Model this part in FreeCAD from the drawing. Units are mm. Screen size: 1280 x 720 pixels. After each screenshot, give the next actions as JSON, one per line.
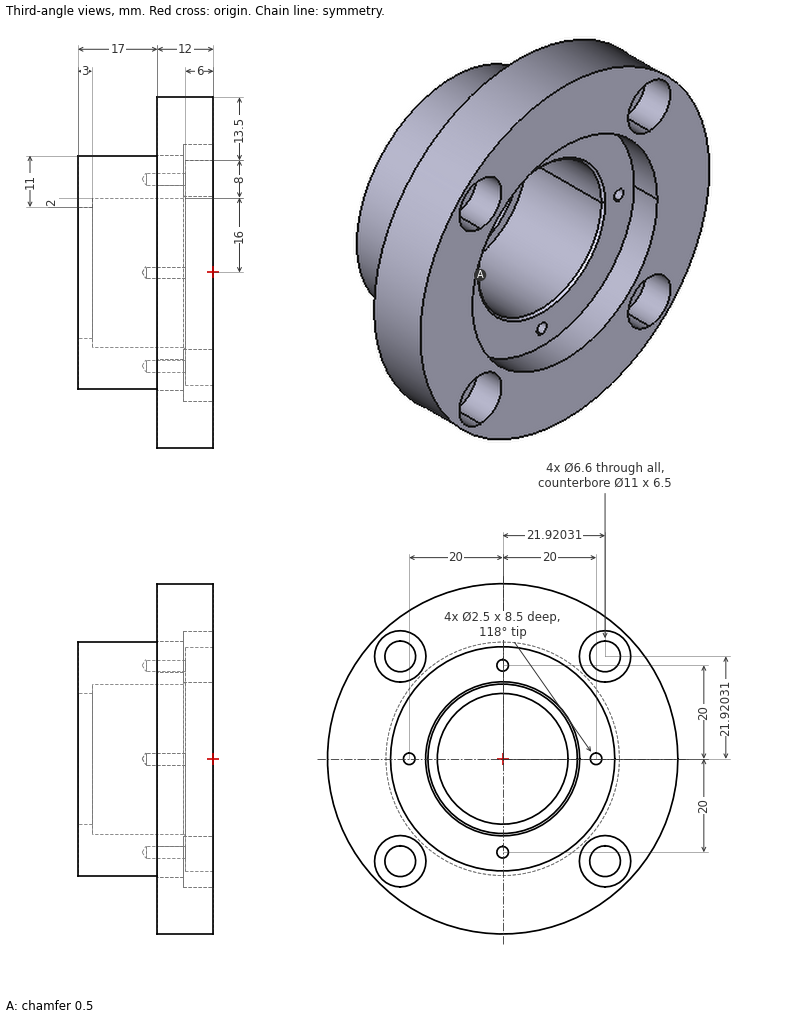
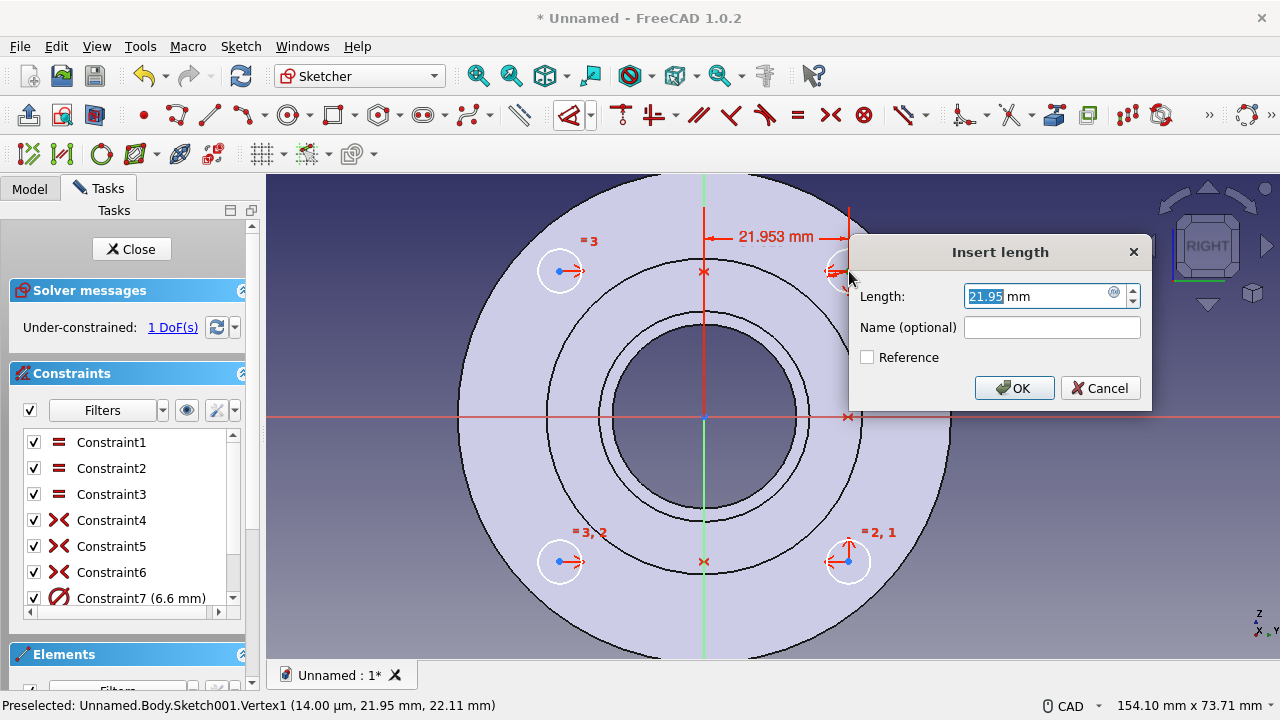
{"action": "type", "text": "21.92031"}
{"action": "key", "text": "Return"}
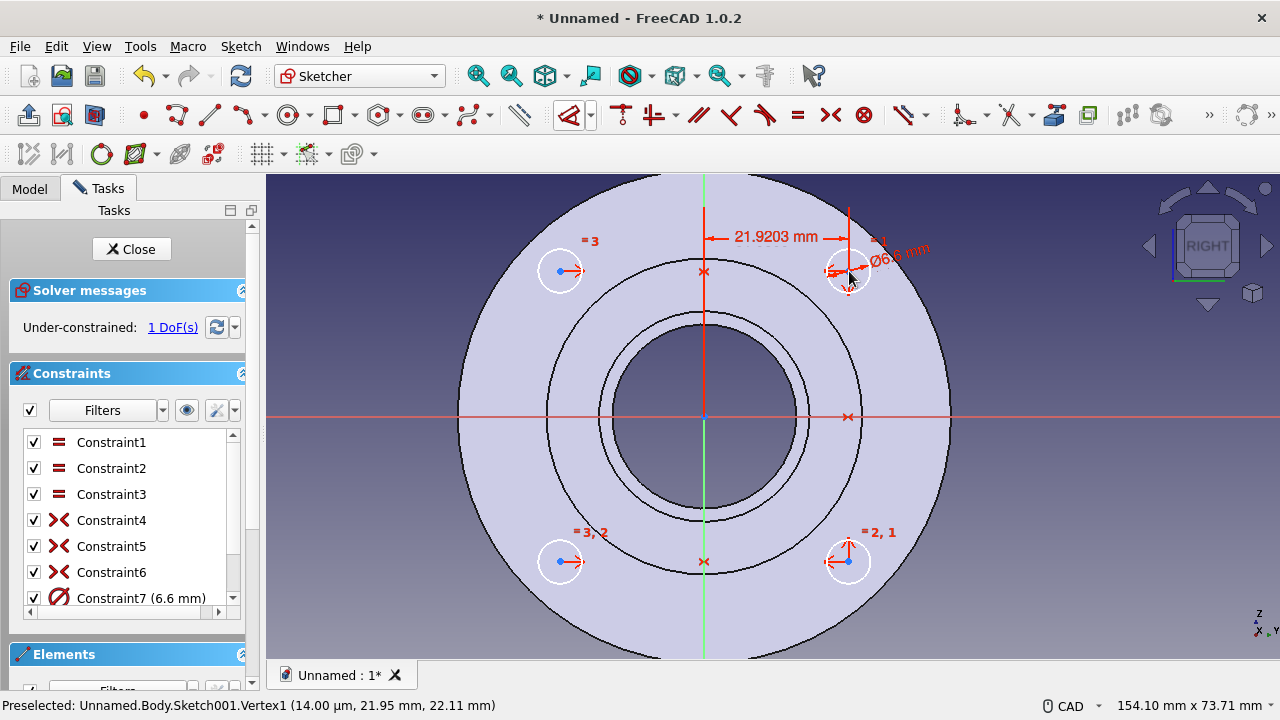
{"action": "left_click", "coordinate": [849, 271]}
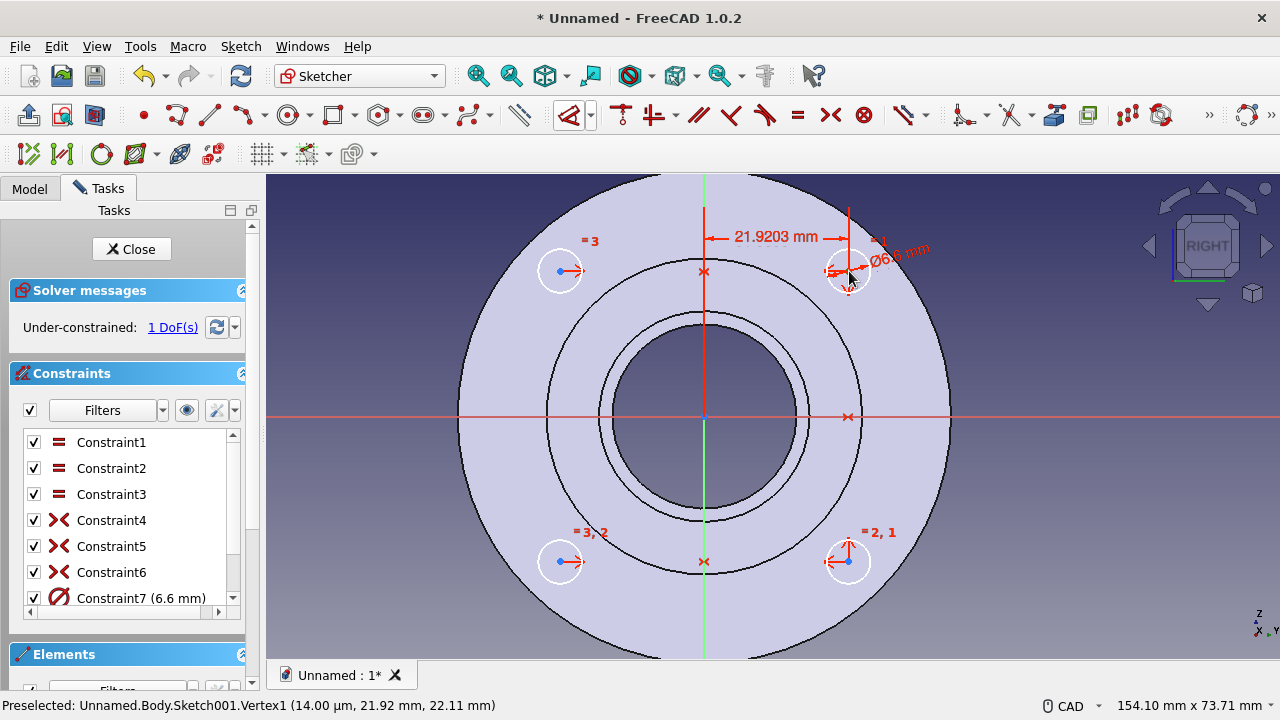
{"action": "key", "text": "i"}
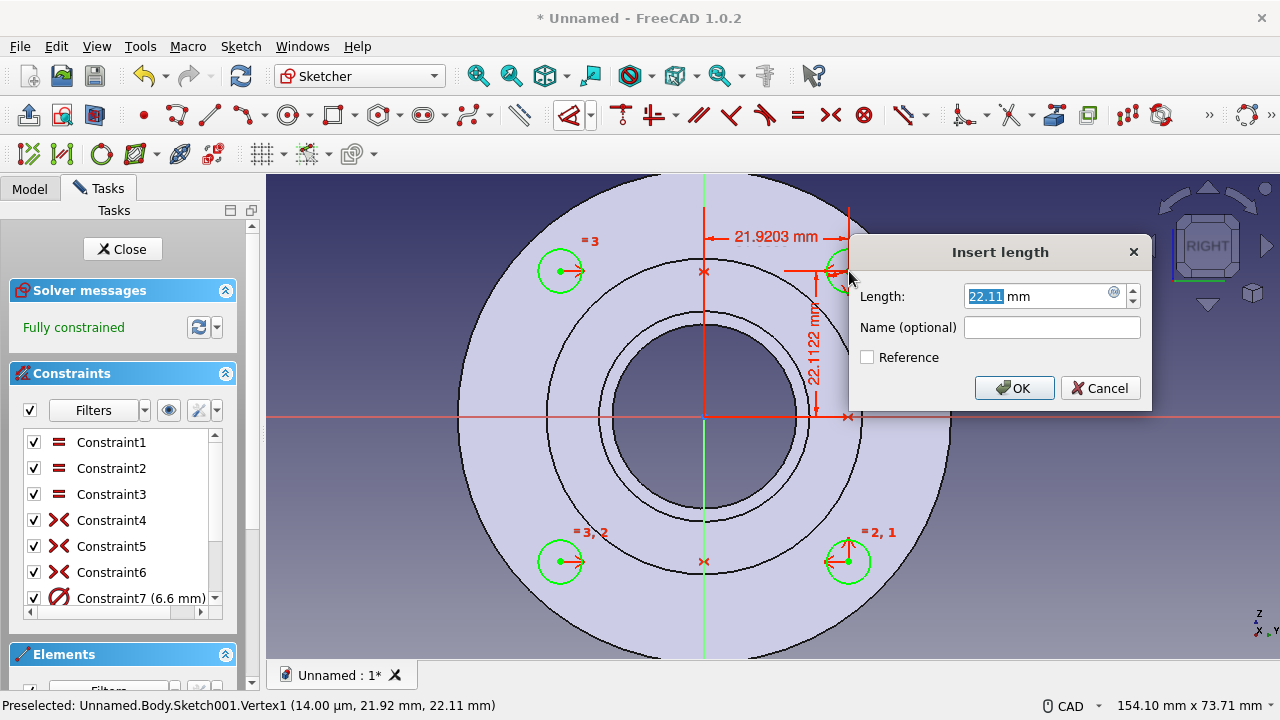
{"action": "type", "text": "21.92031"}
{"action": "key", "text": "Return"}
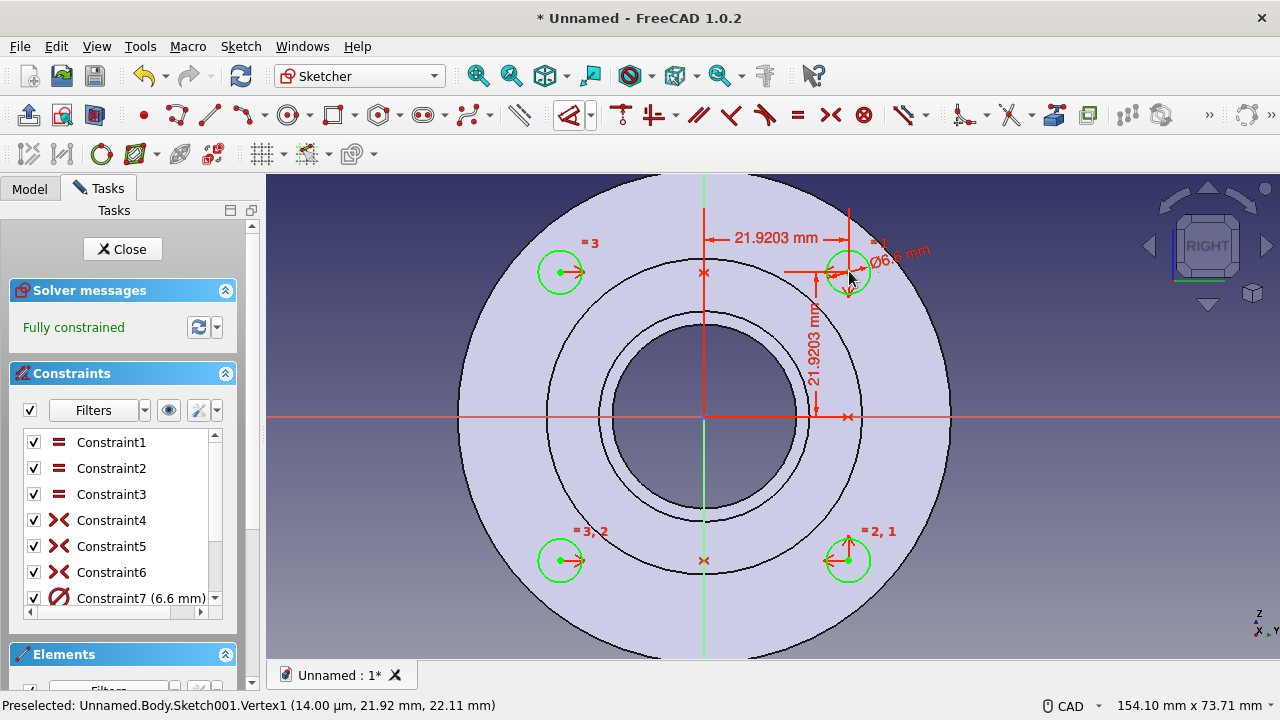
{"action": "left_click", "coordinate": [123, 249]}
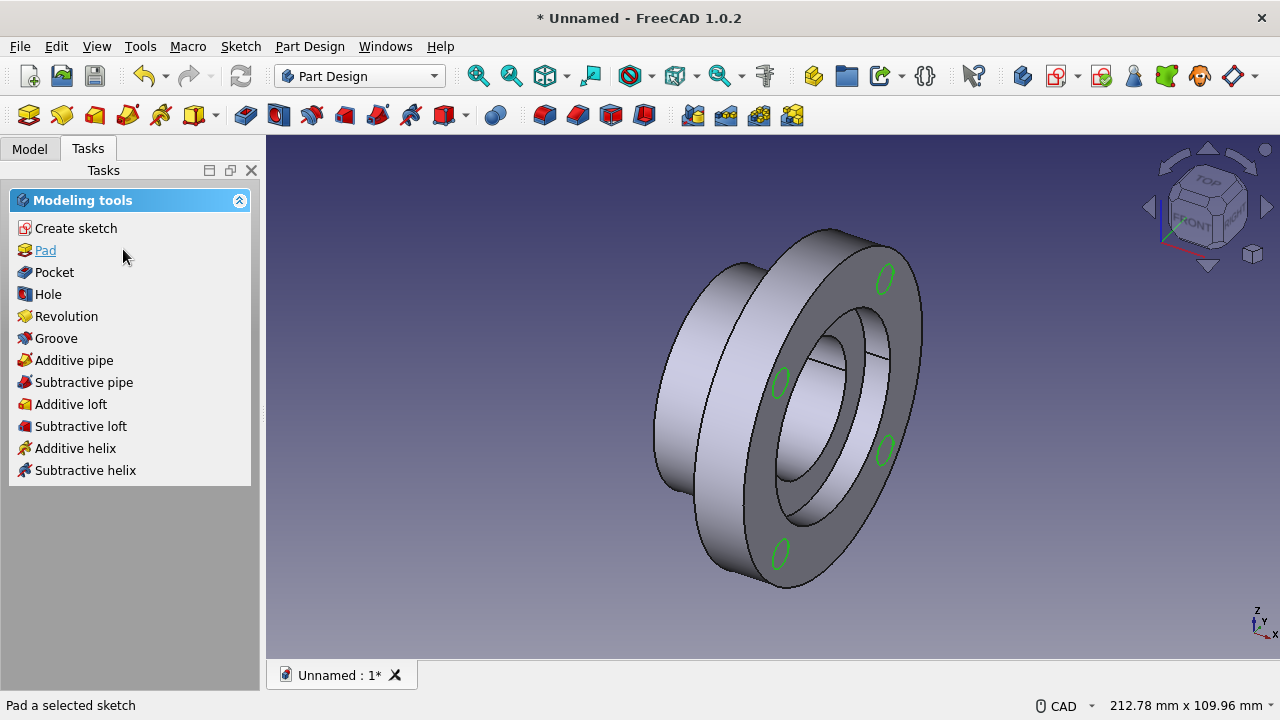
{"action": "left_click", "coordinate": [279, 116]}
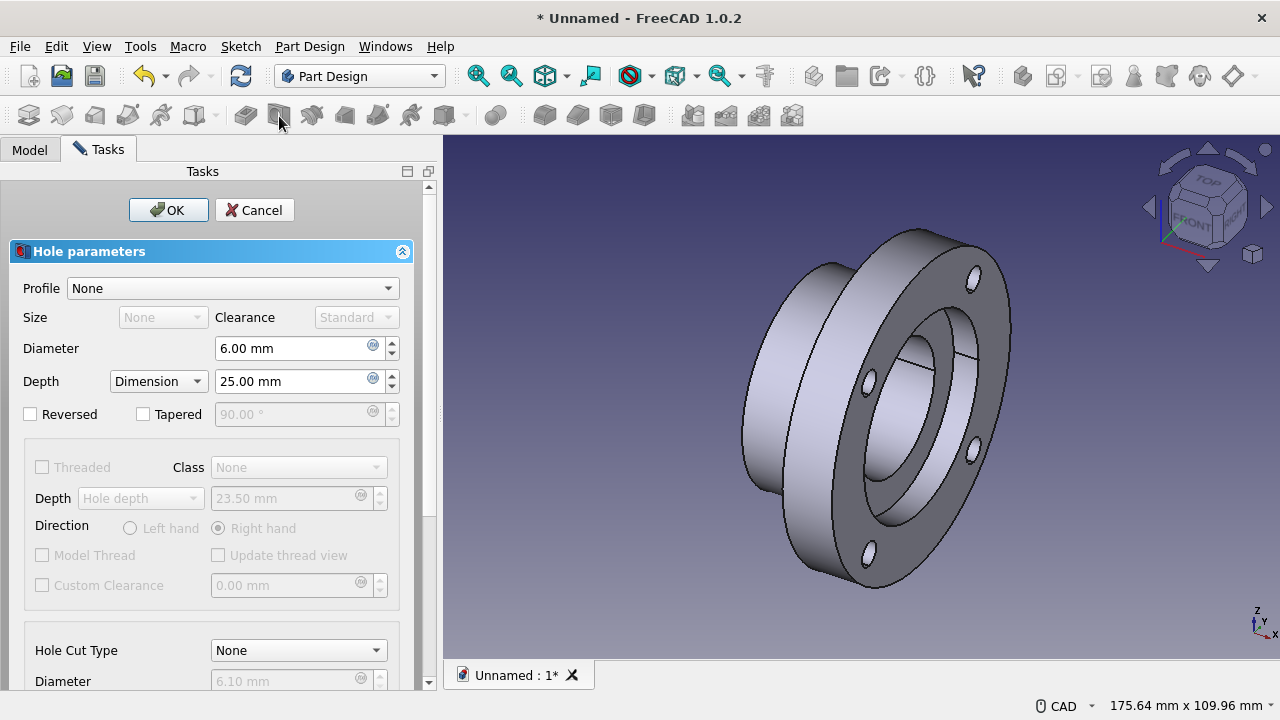
{"action": "triple_click", "coordinate": [300, 348]}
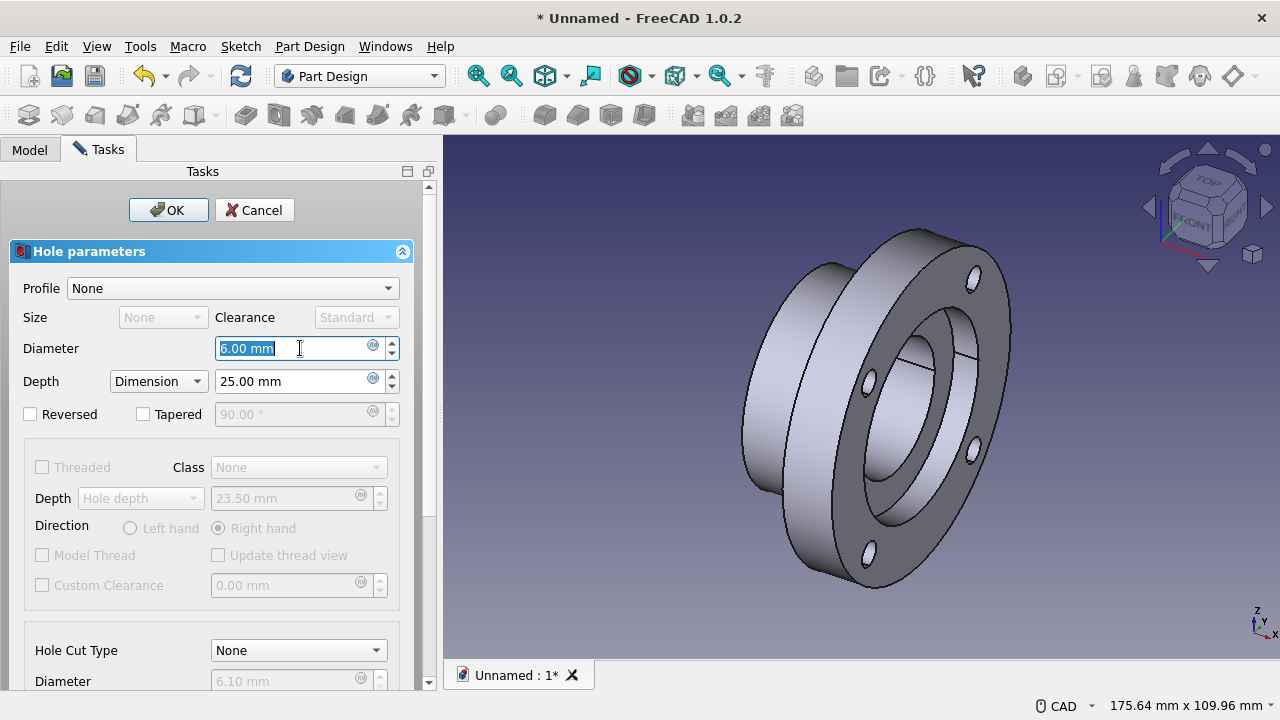
{"action": "type", "text": "6.6"}
{"action": "key", "text": "Tab"}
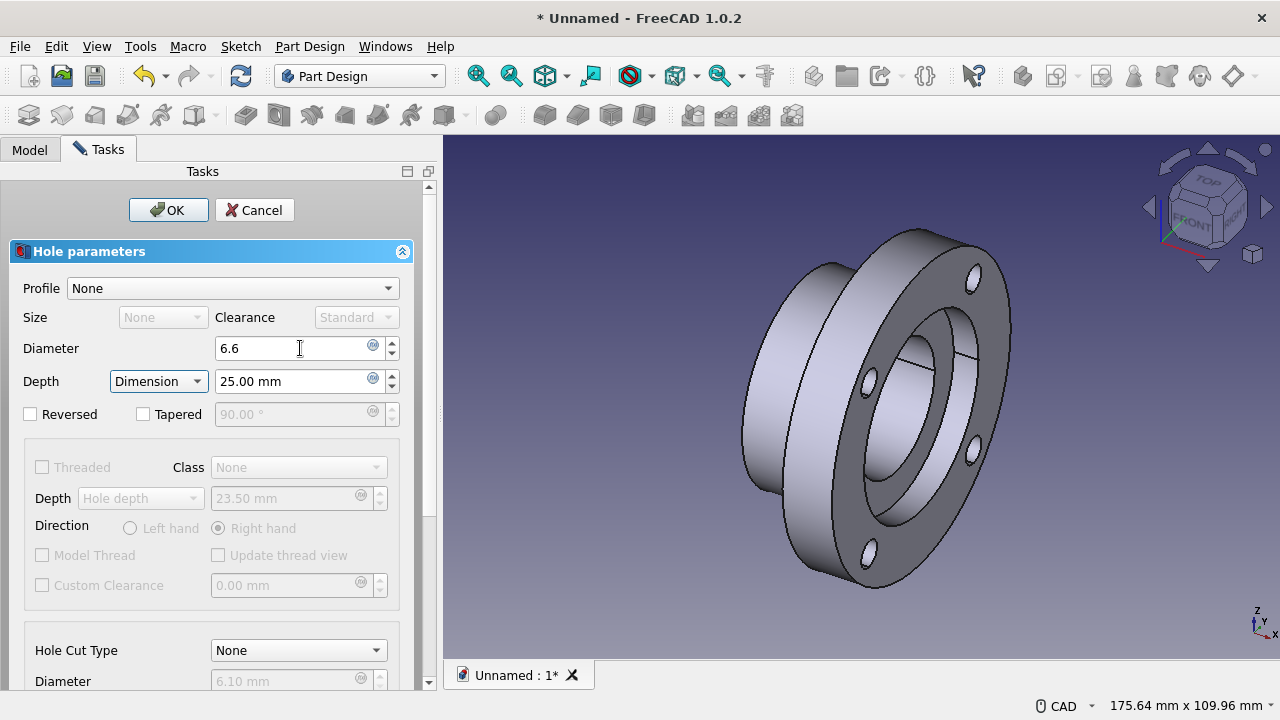
{"action": "left_click", "coordinate": [160, 382]}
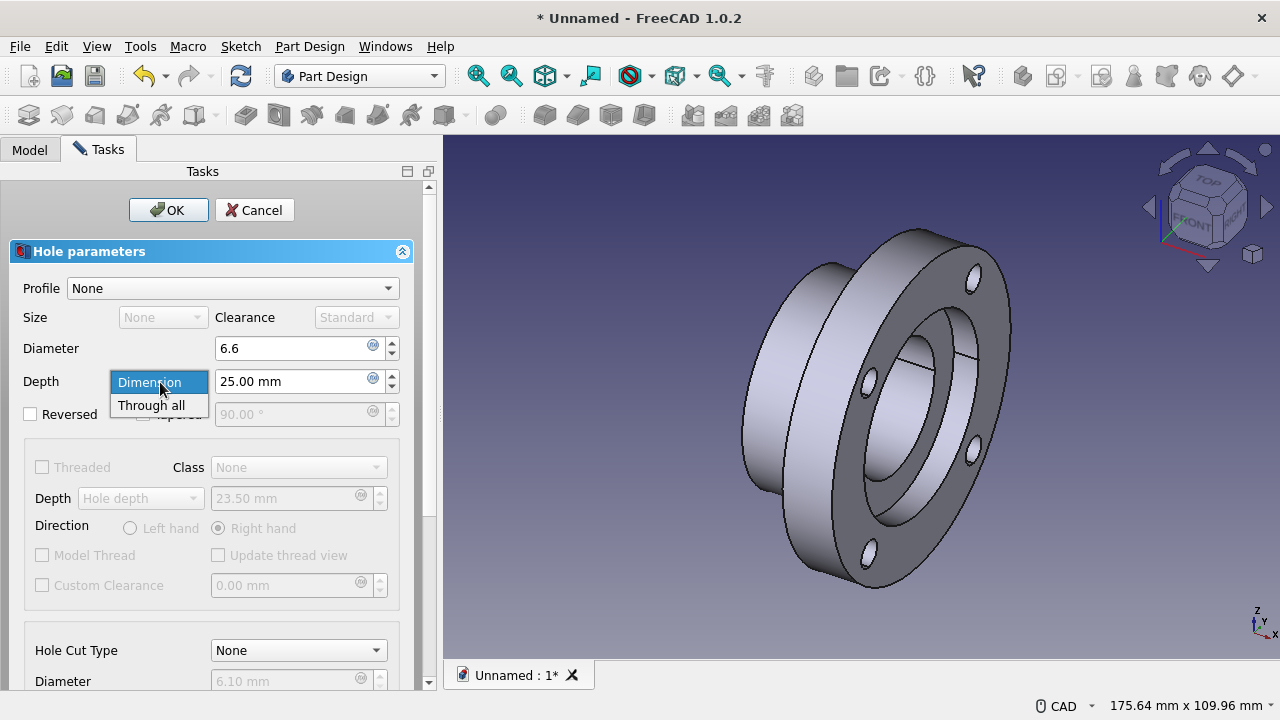
{"action": "left_click", "coordinate": [158, 406]}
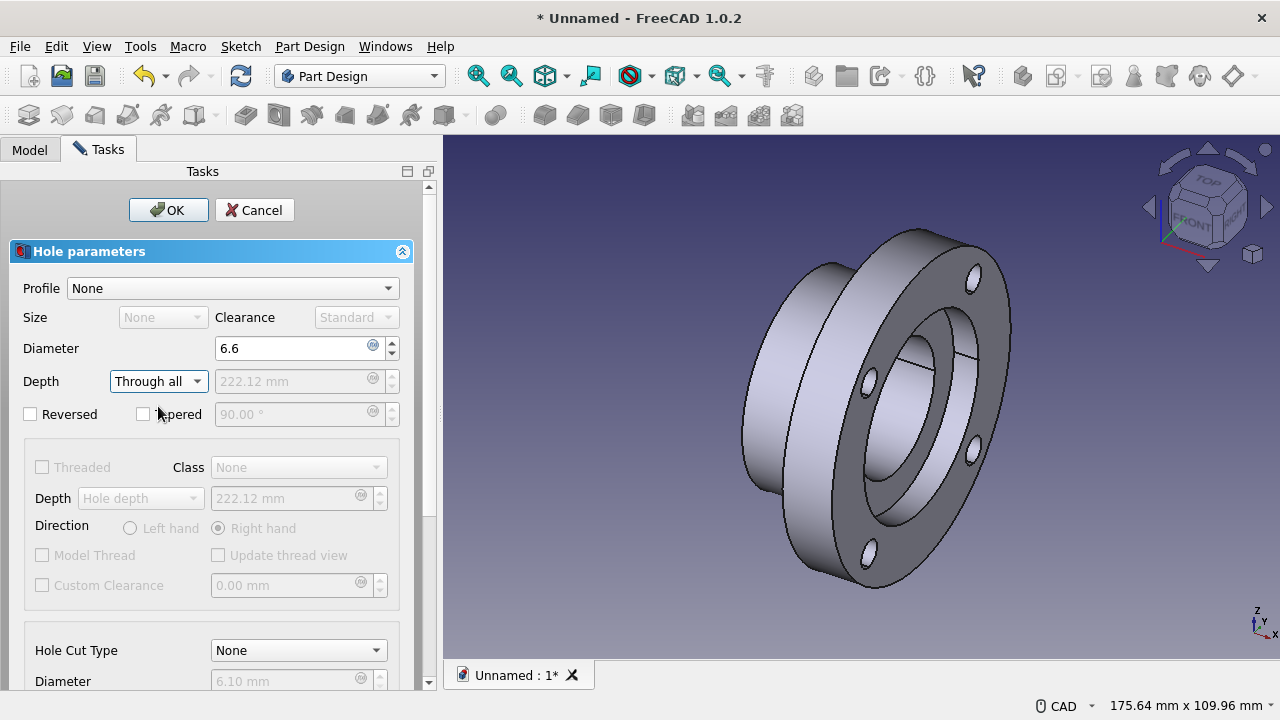
{"action": "left_click", "coordinate": [300, 650]}